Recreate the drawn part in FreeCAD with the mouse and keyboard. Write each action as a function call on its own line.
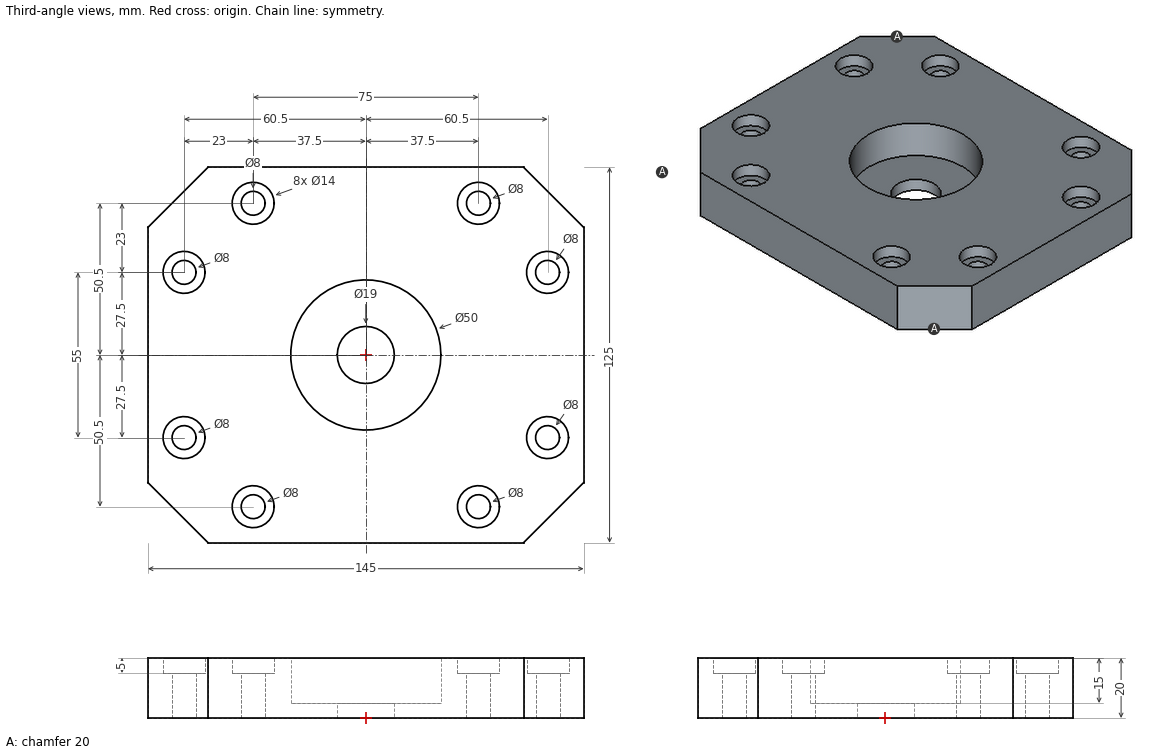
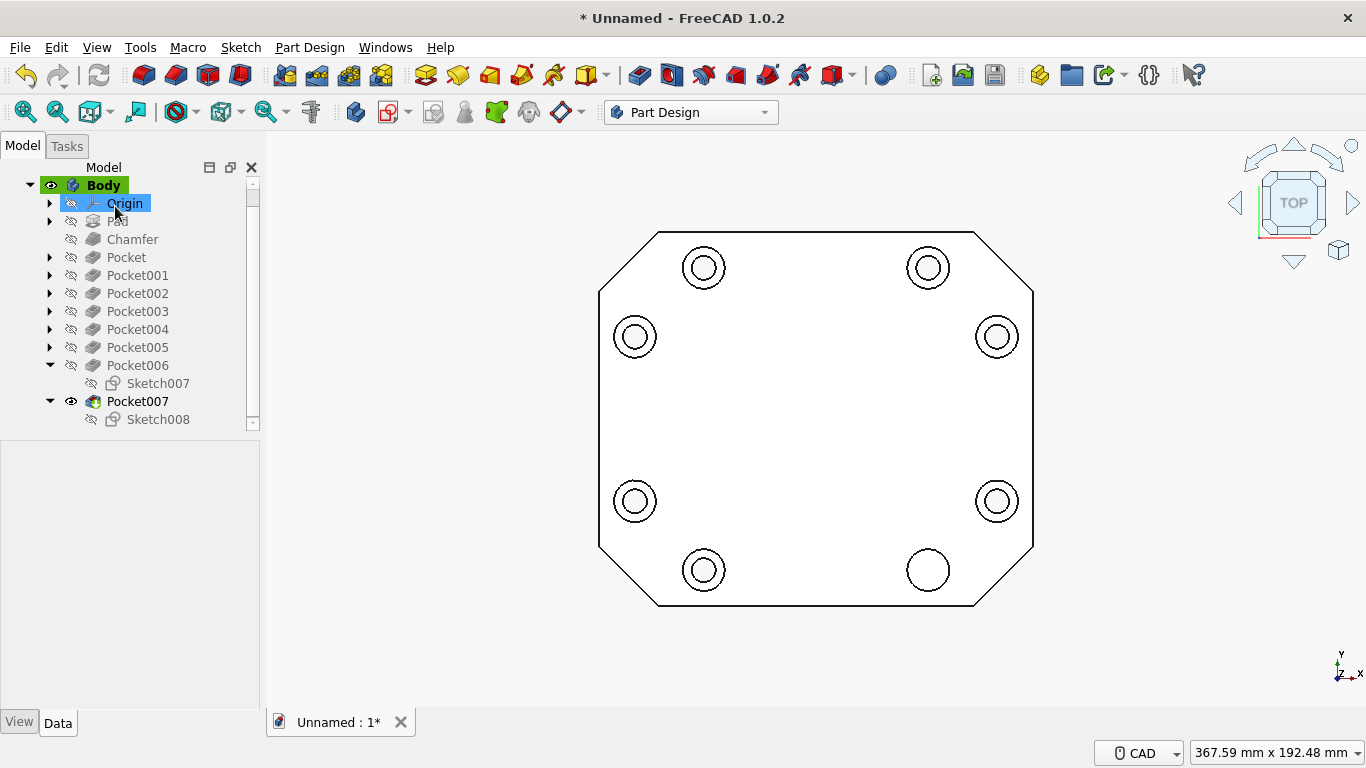
click(928, 569)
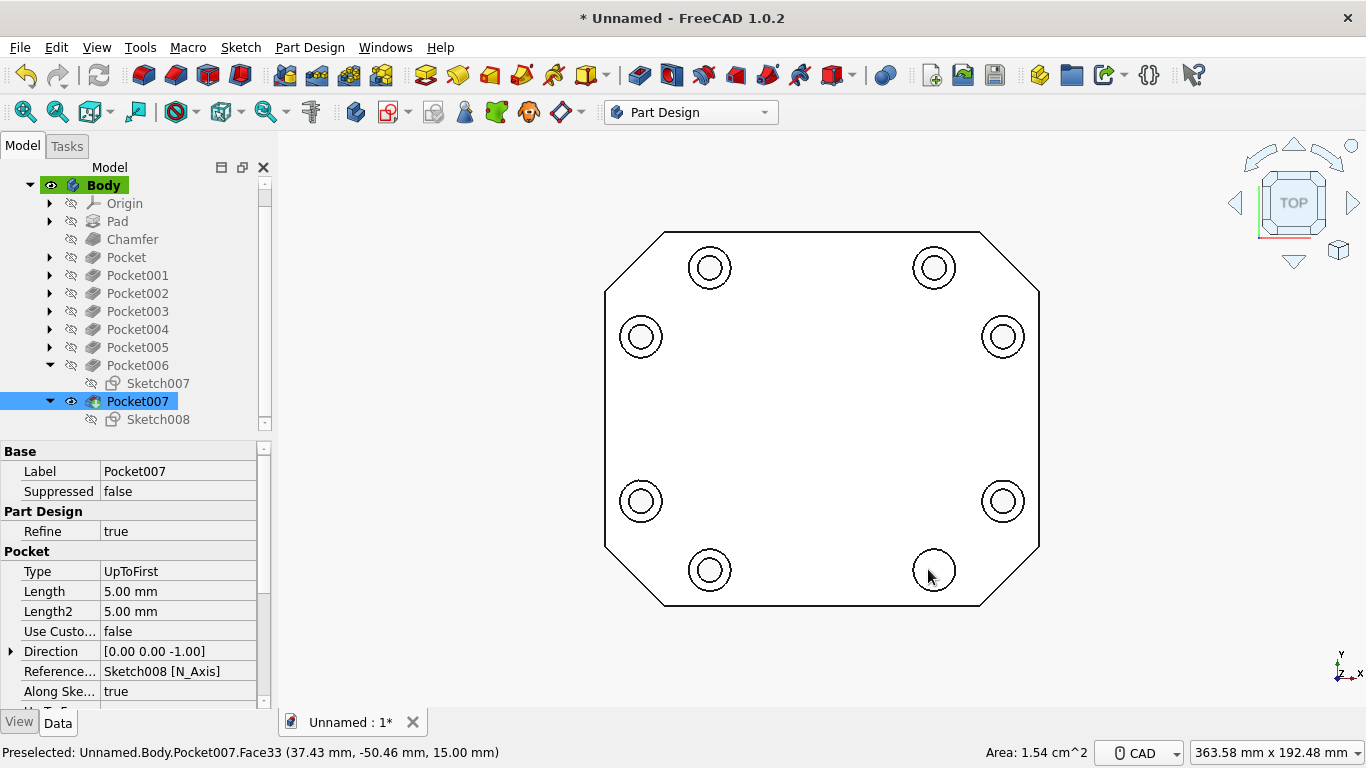
click(388, 112)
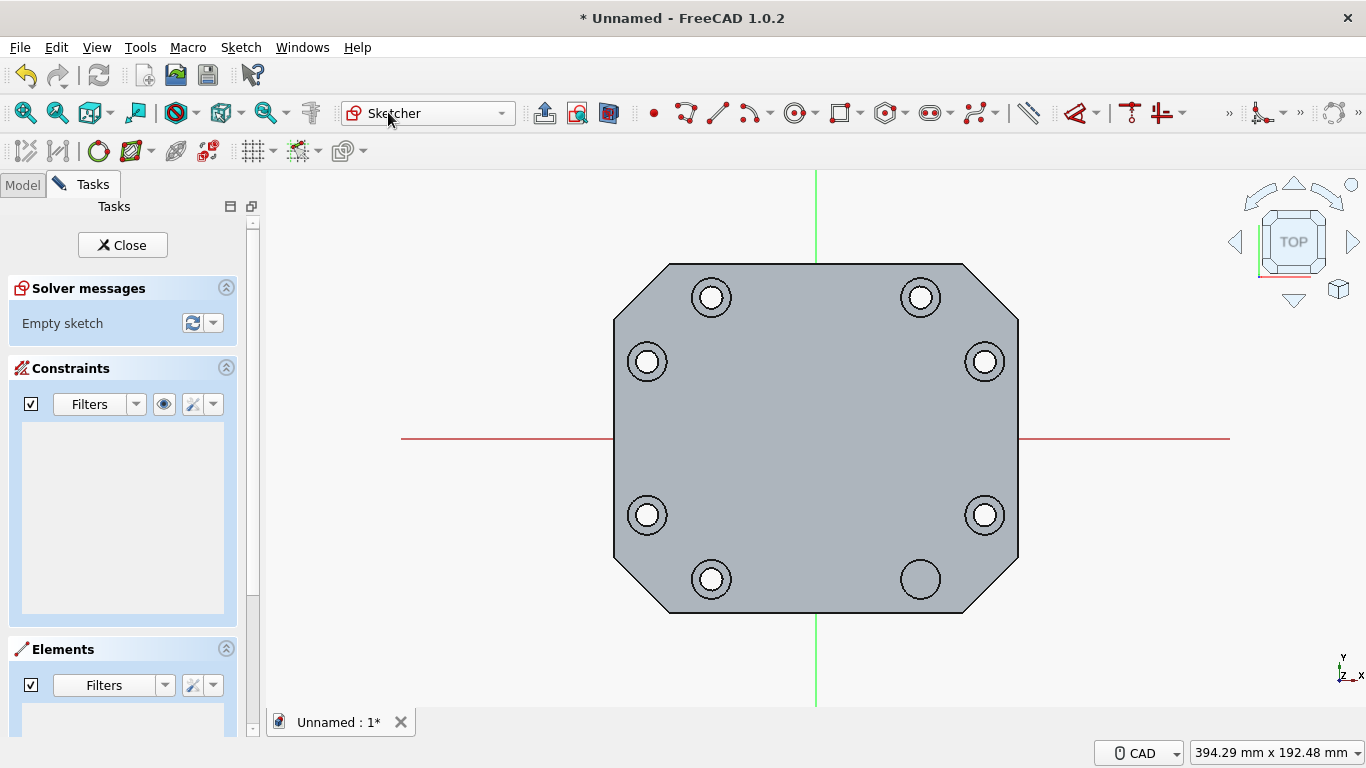
click(610, 114)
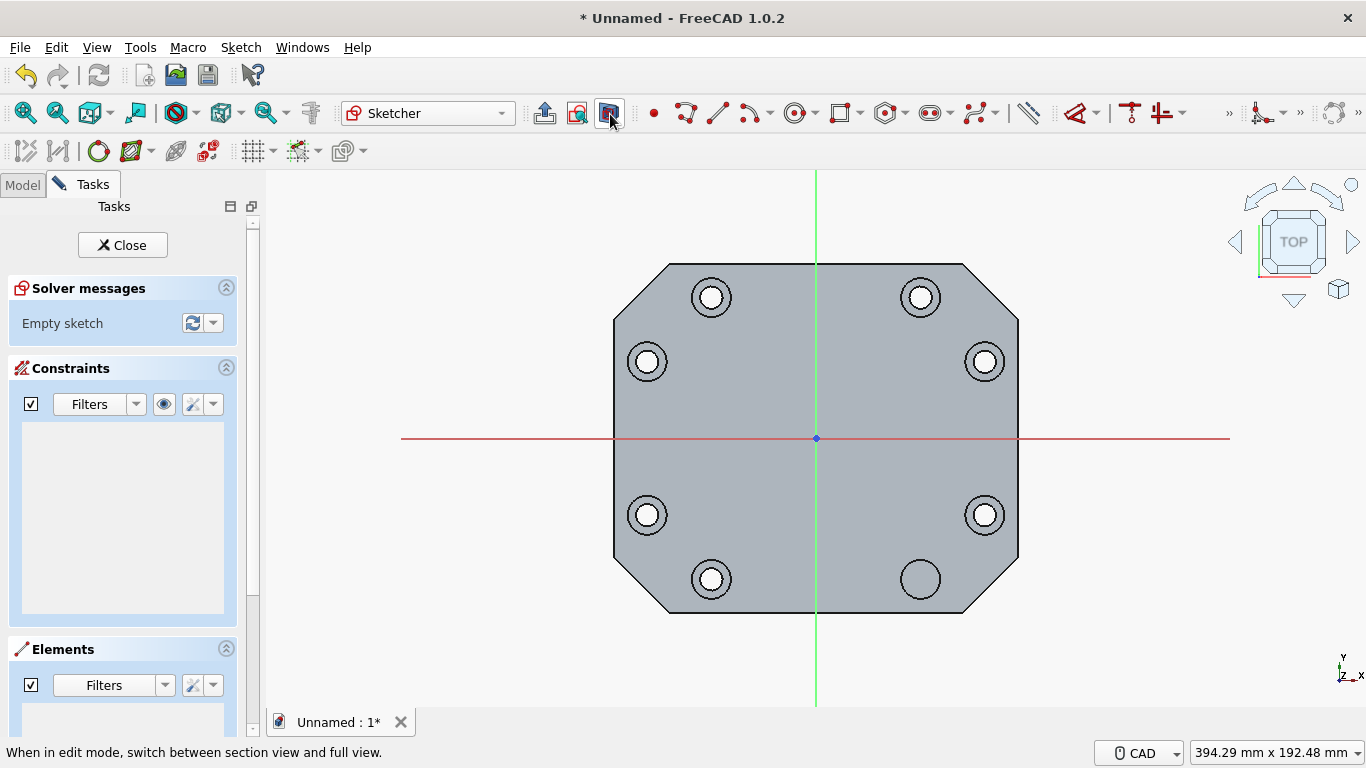
scroll(932, 589, up, 14)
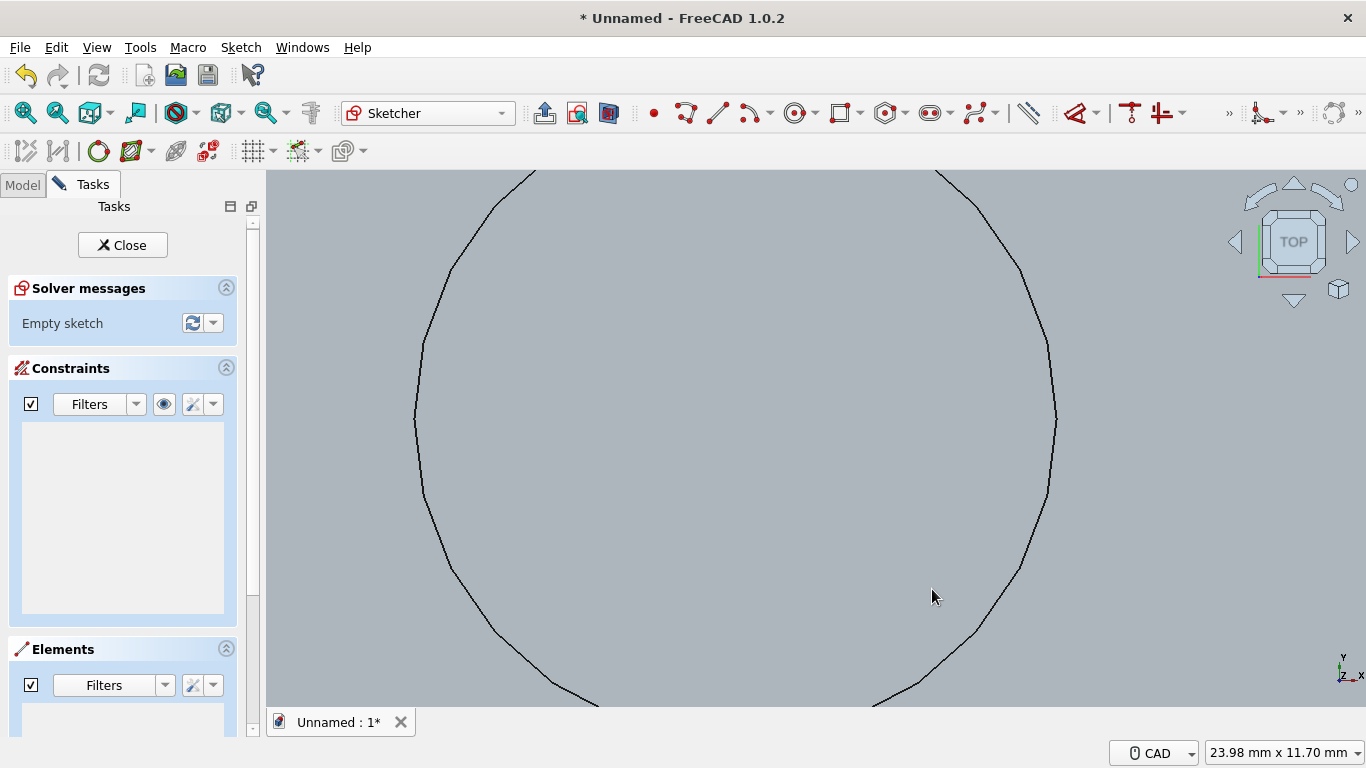
click(796, 114)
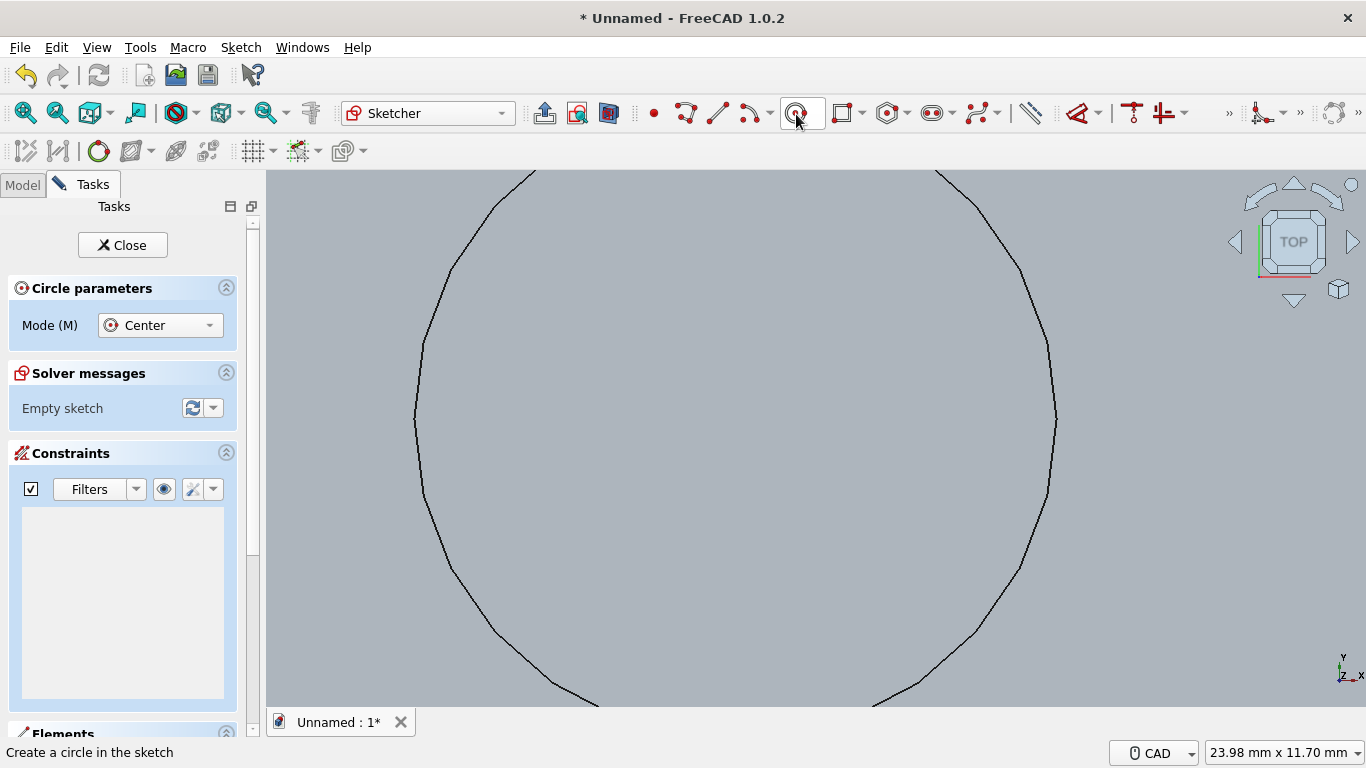
click(735, 419)
click(865, 289)
key(Escape)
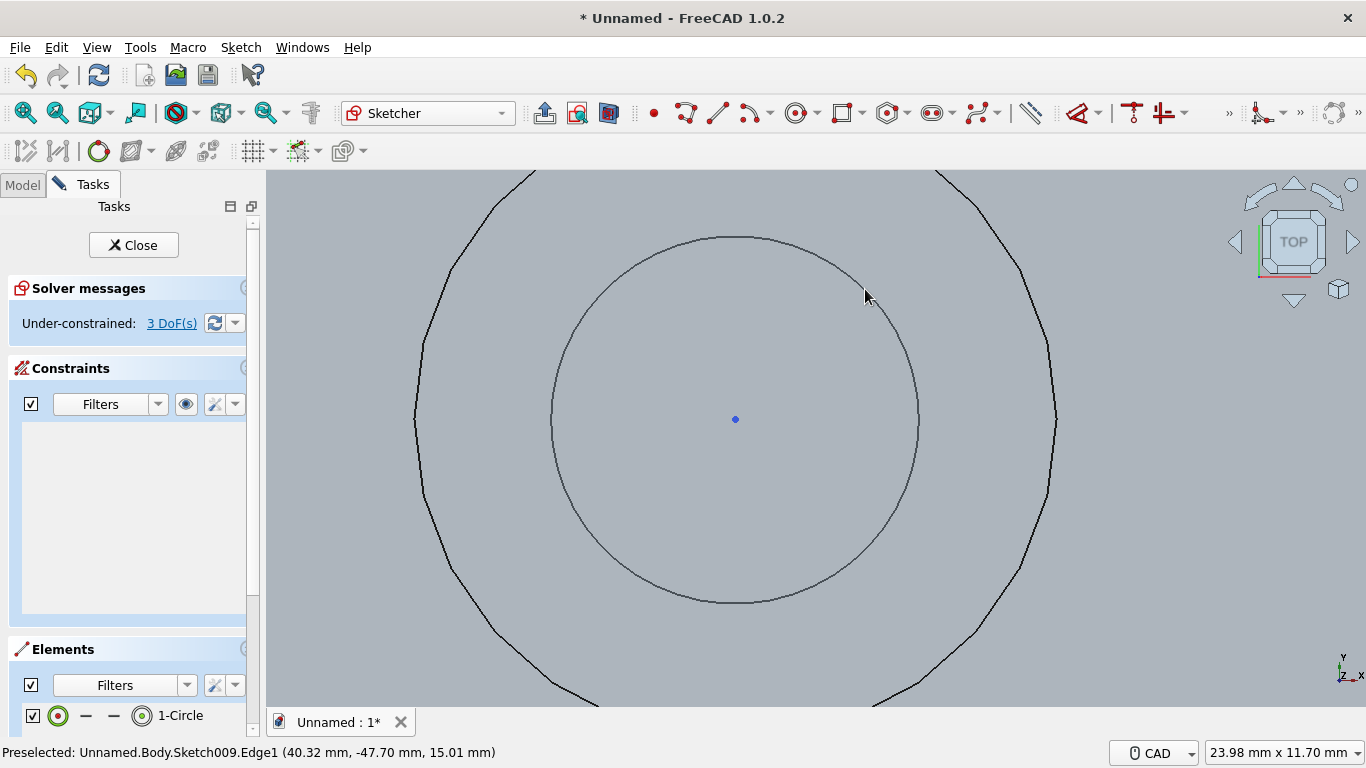
click(1078, 114)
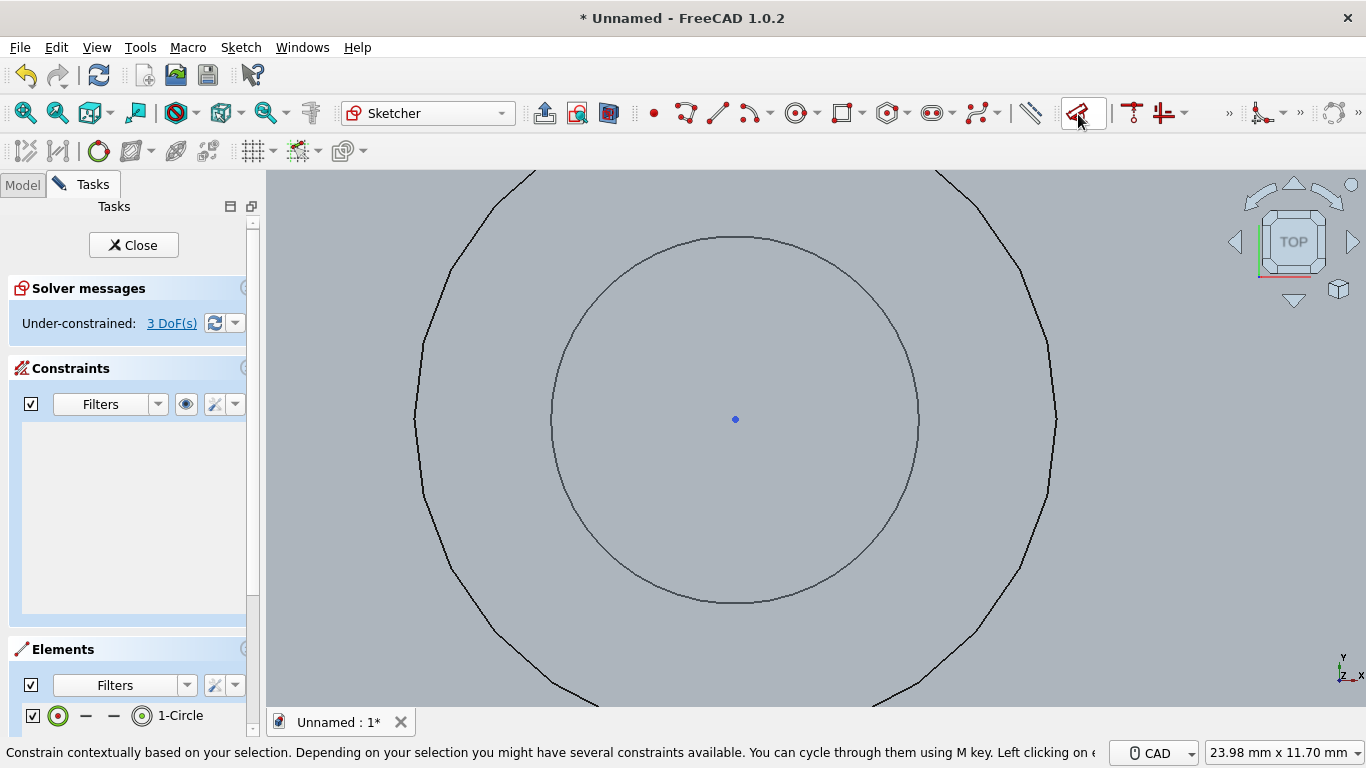
click(865, 290)
click(888, 267)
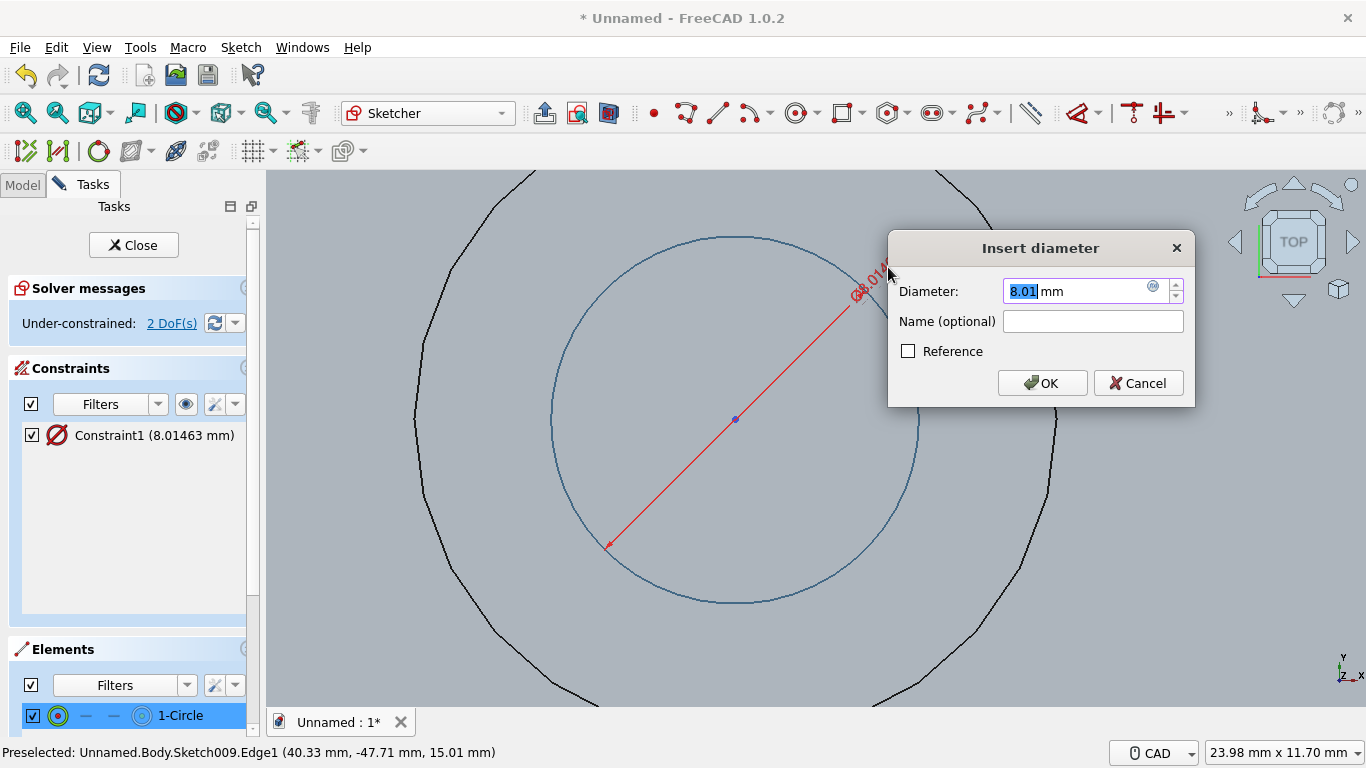
text(8)
key(Return)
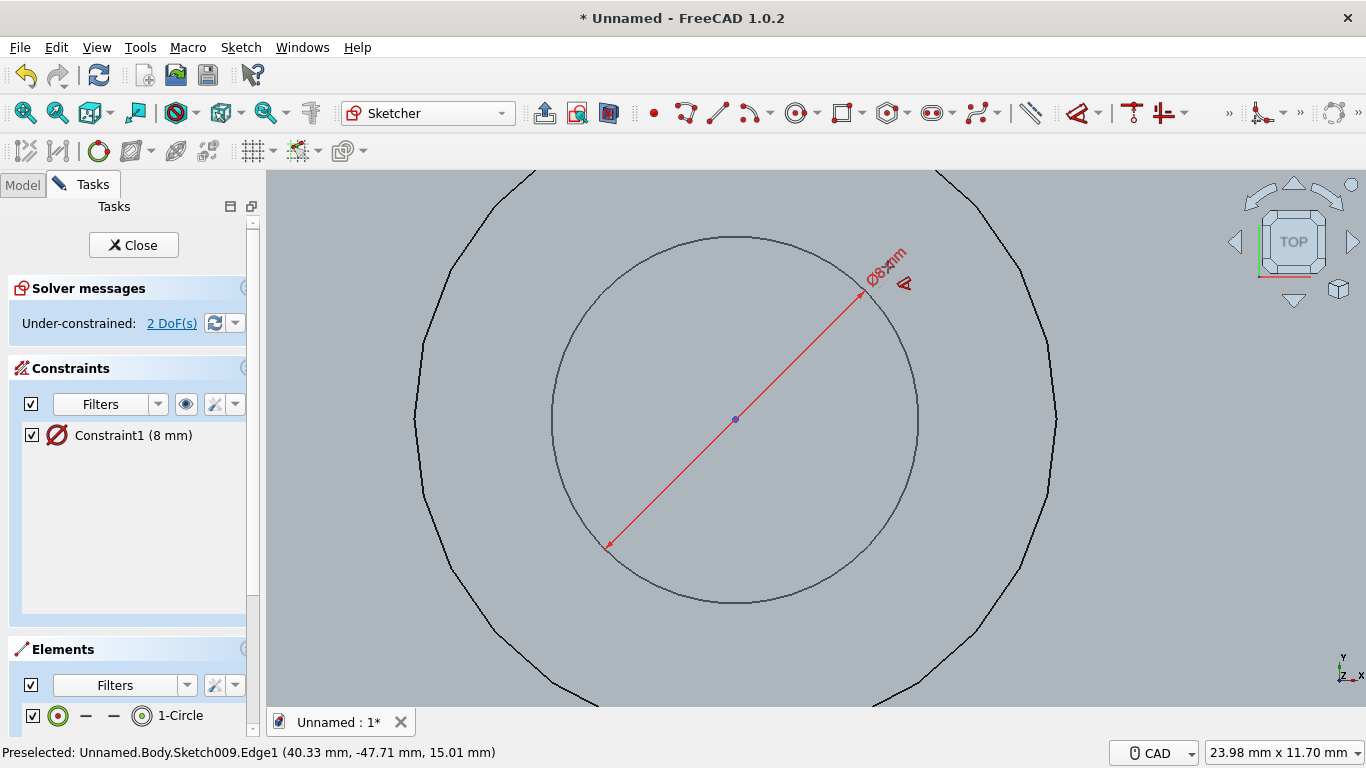
click(735, 420)
click(514, 454)